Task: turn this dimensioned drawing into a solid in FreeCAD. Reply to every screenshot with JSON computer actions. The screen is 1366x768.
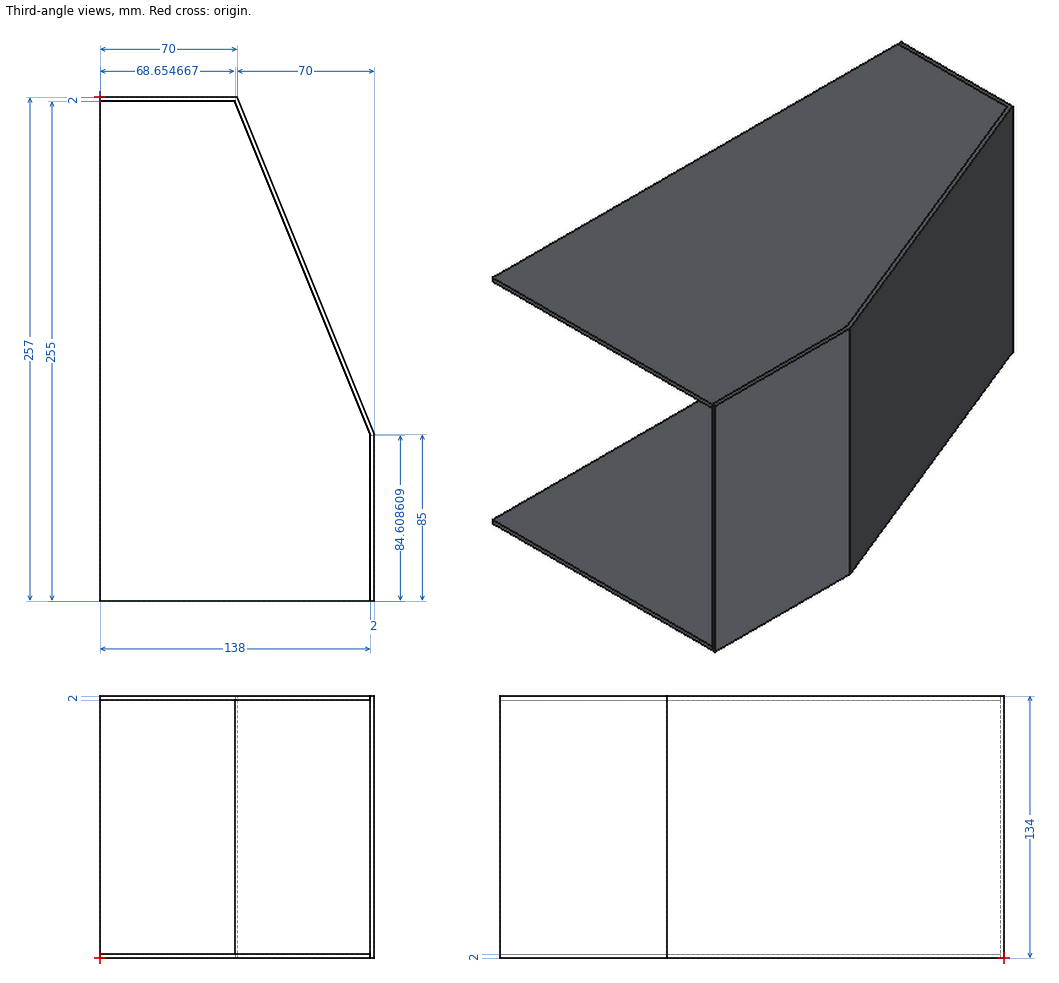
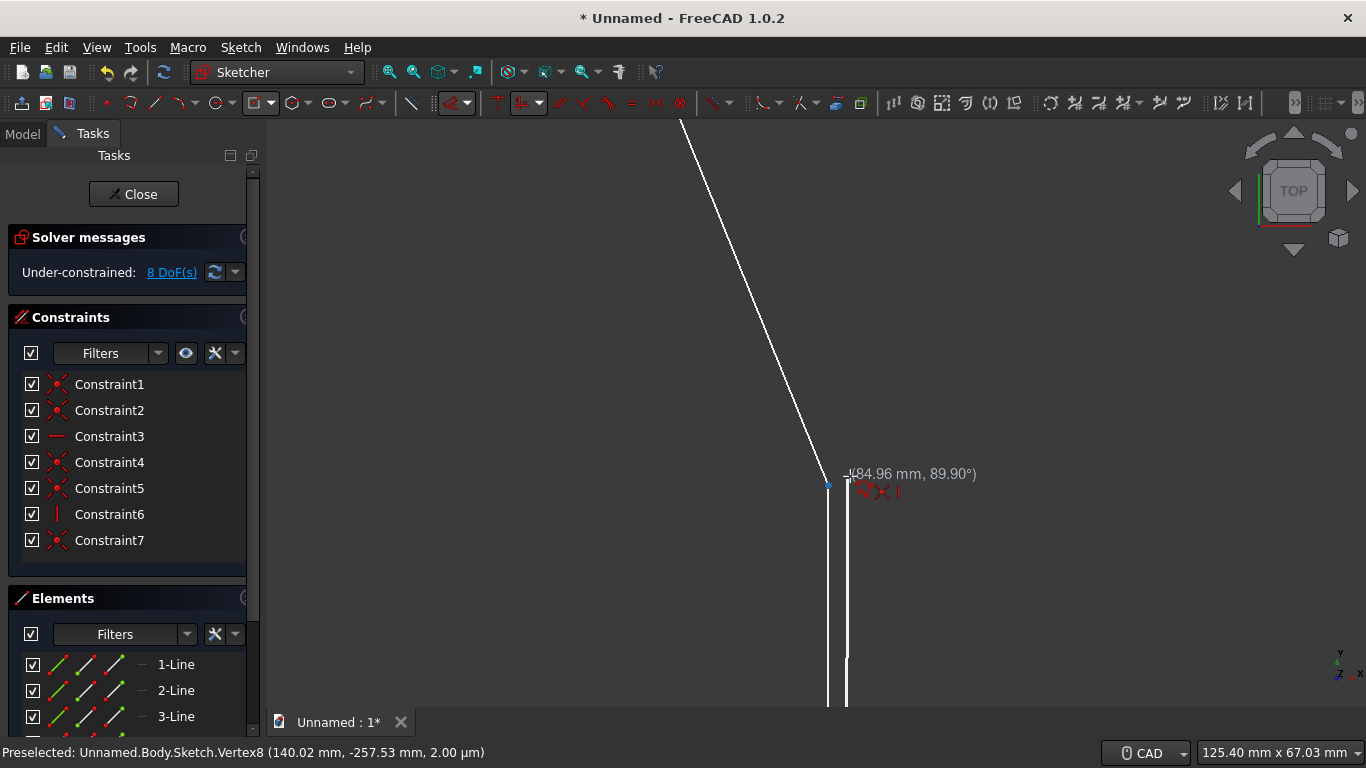
{"action": "left_click", "coordinate": [846, 475]}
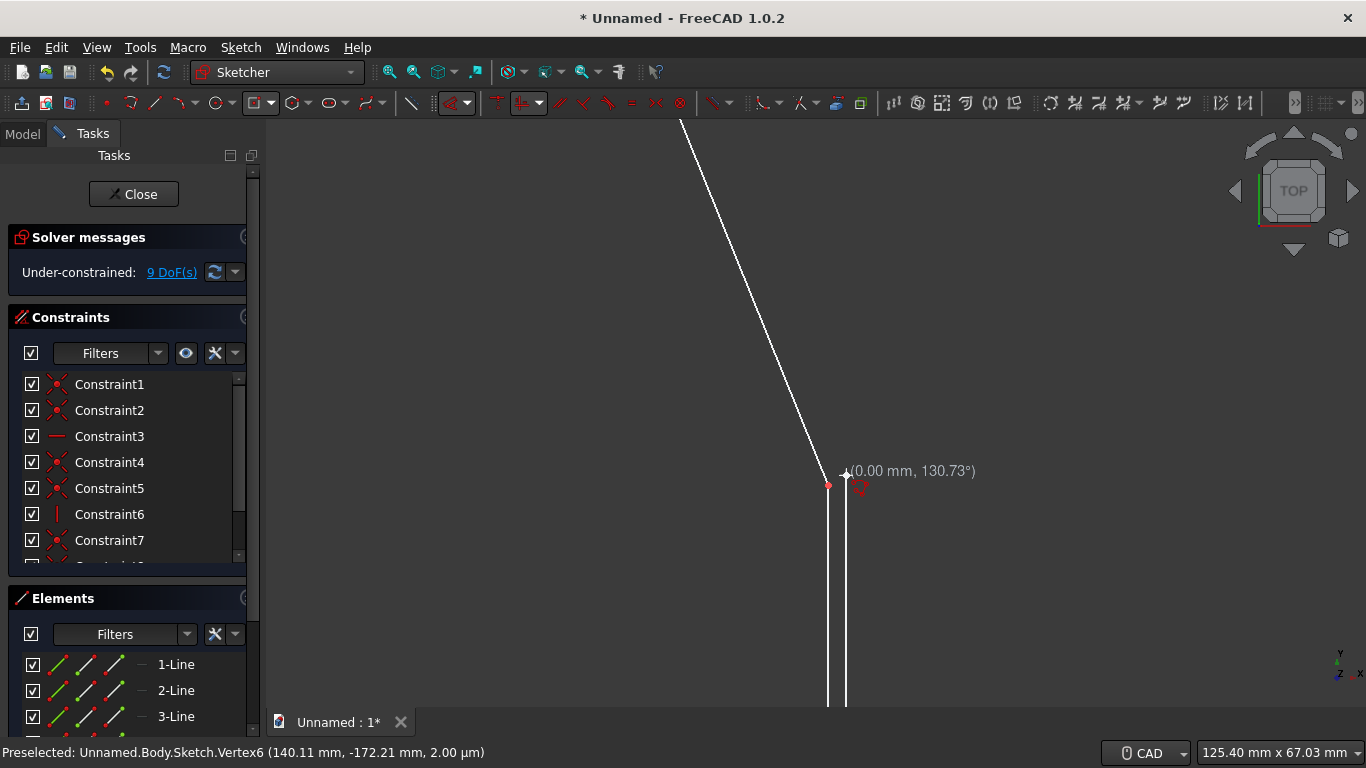
{"action": "scroll", "coordinate": [850, 476], "scroll_direction": "down", "scroll_amount": 9}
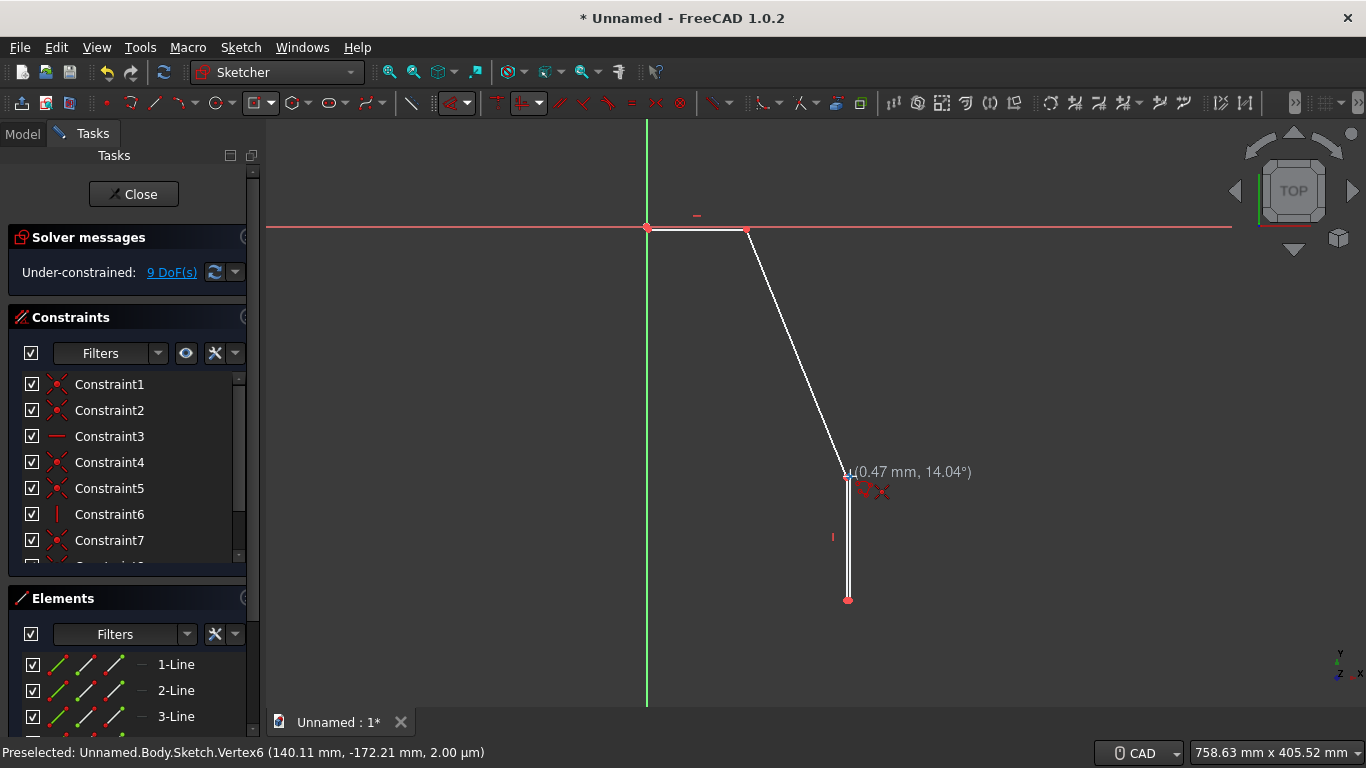
{"action": "scroll", "coordinate": [748, 227], "scroll_direction": "up", "scroll_amount": 8}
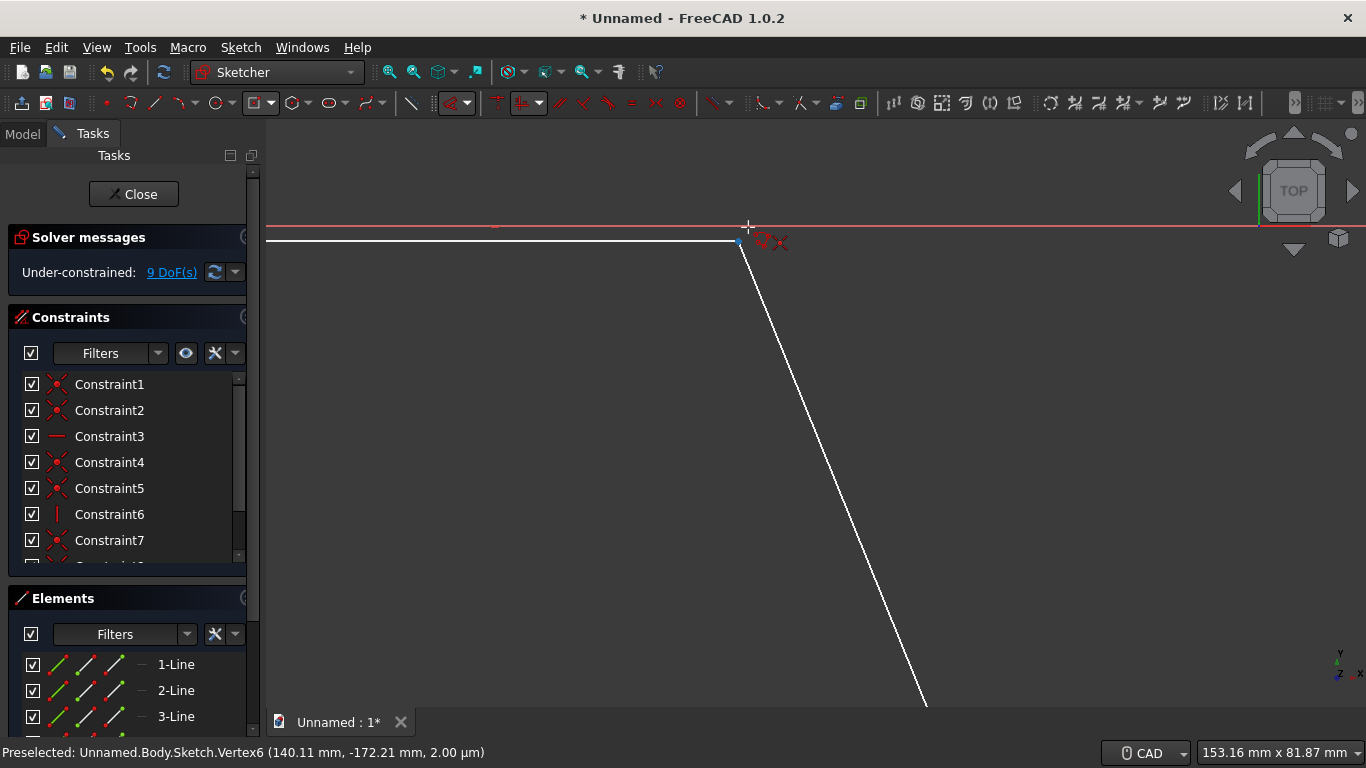
{"action": "left_click", "coordinate": [748, 235]}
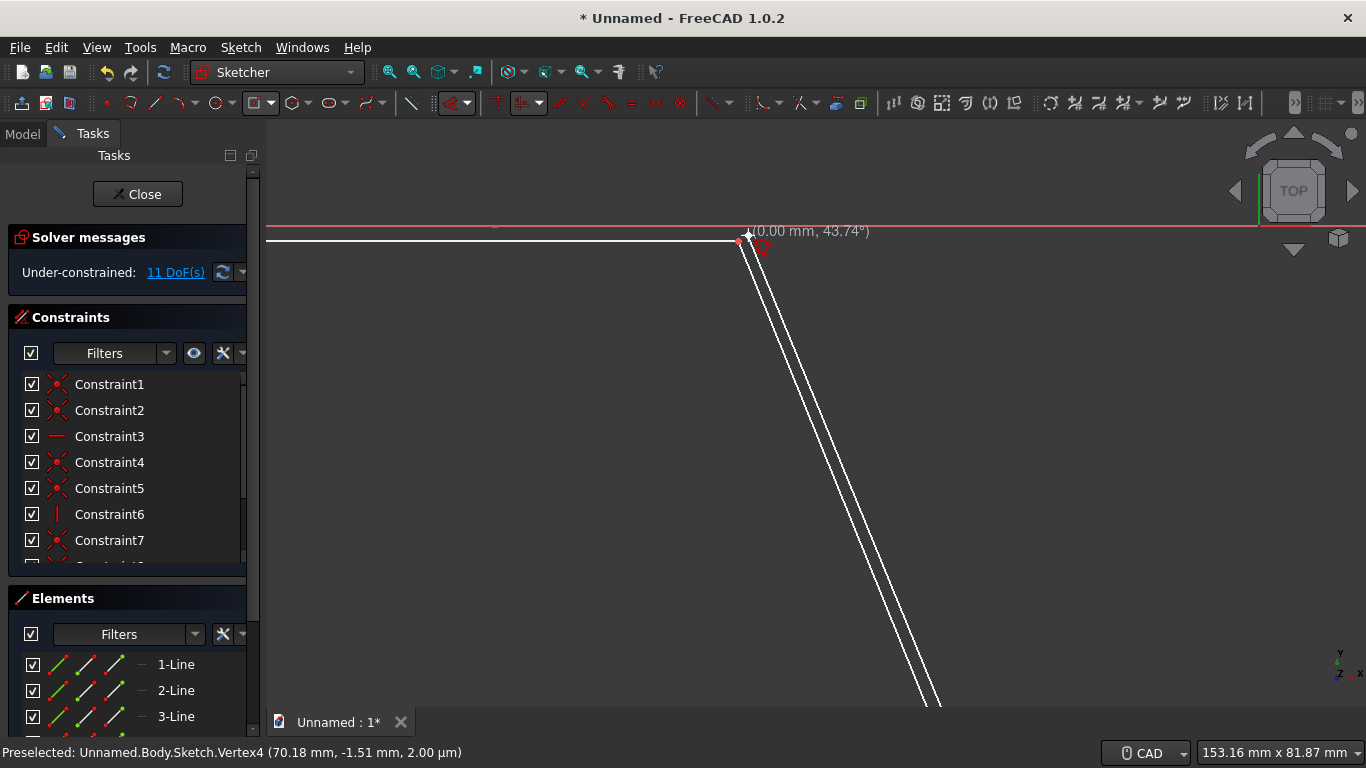
{"action": "scroll", "coordinate": [747, 227], "scroll_direction": "down", "scroll_amount": 8}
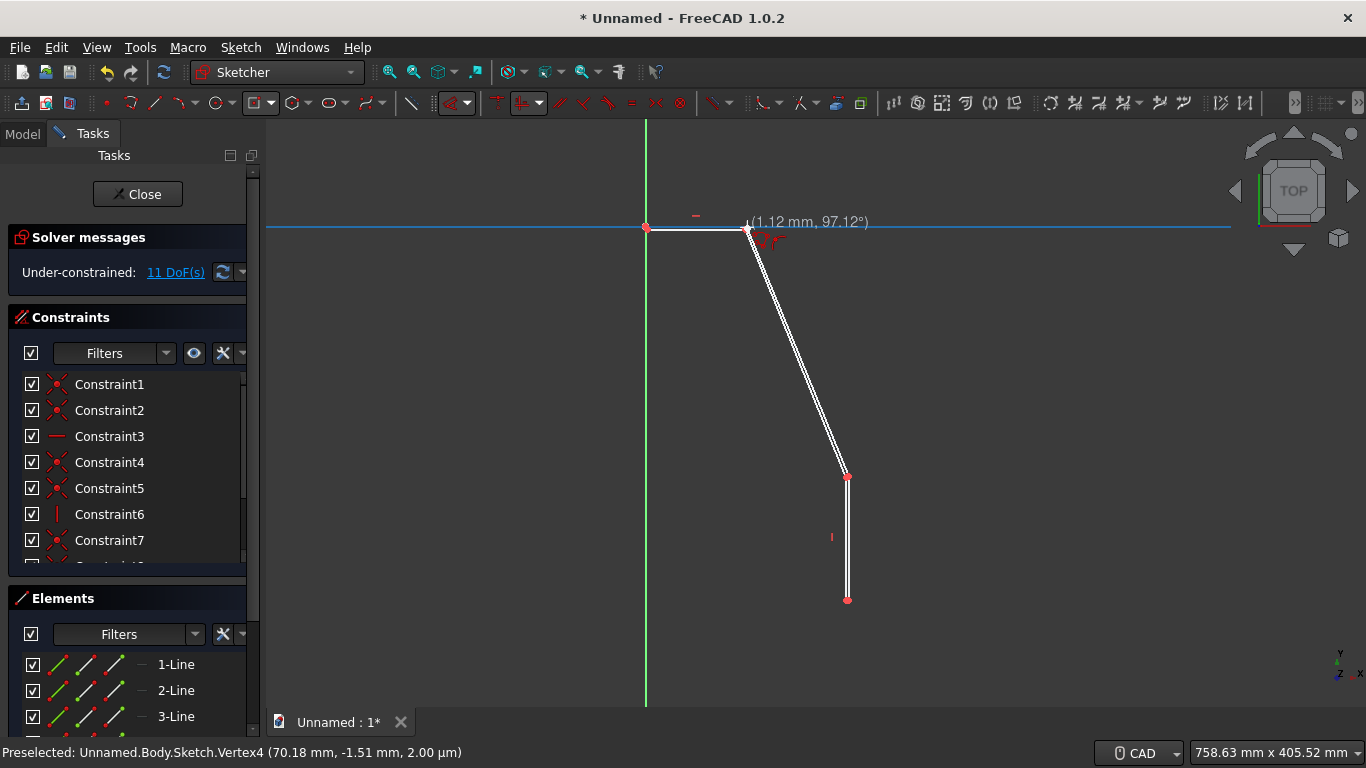
{"action": "scroll", "coordinate": [646, 227], "scroll_direction": "up", "scroll_amount": 12}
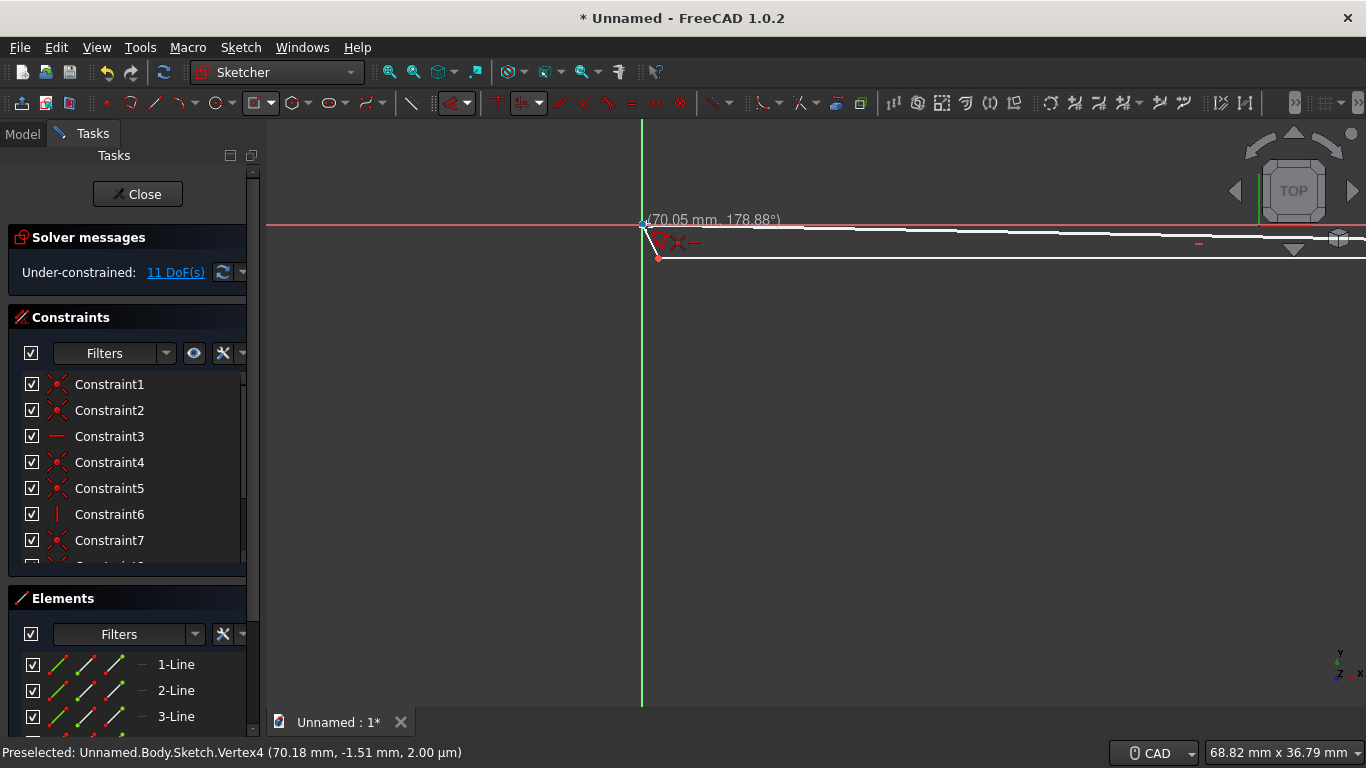
{"action": "left_click", "coordinate": [642, 225]}
{"action": "key", "text": "Escape"}
{"action": "key", "text": "Escape"}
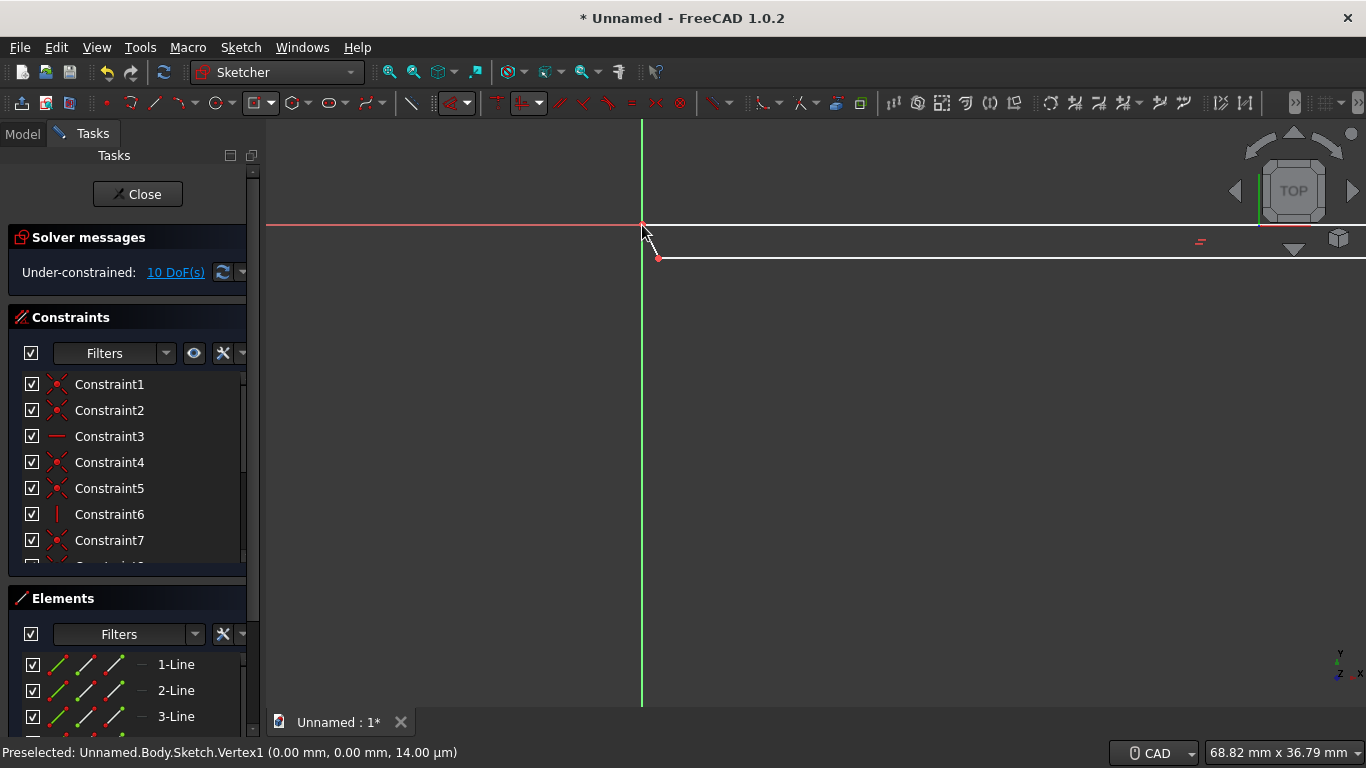
{"action": "scroll", "coordinate": [654, 248], "scroll_direction": "up", "scroll_amount": 2}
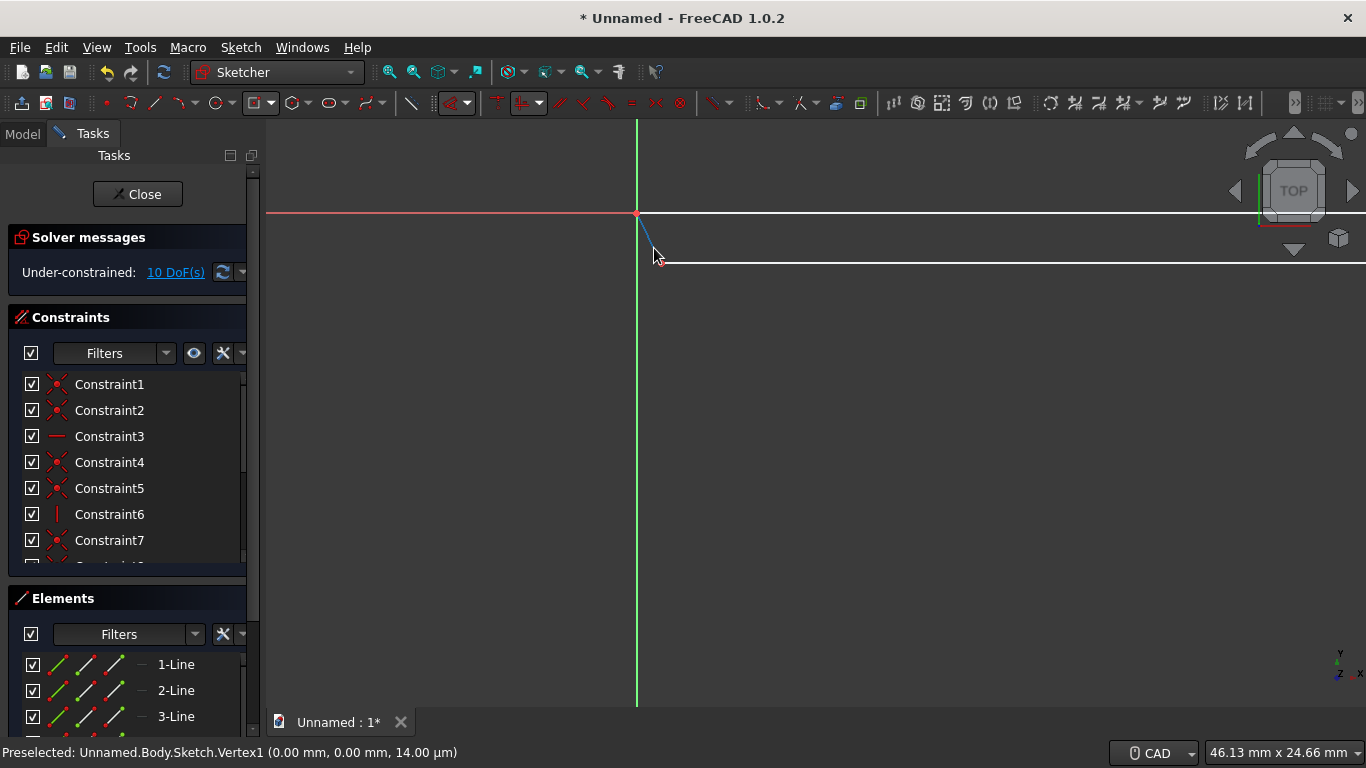
{"action": "left_click", "coordinate": [654, 248]}